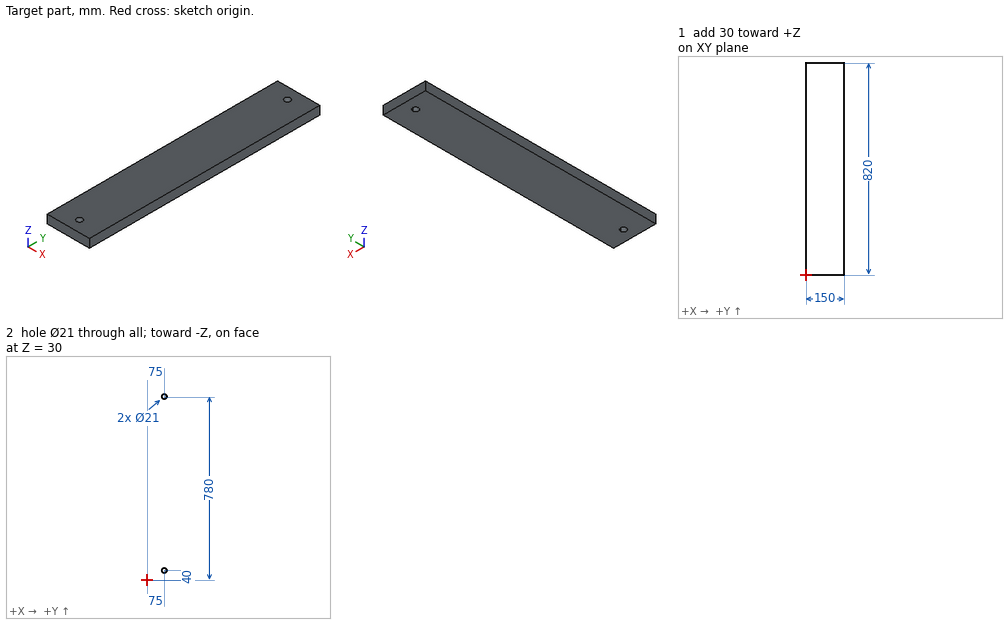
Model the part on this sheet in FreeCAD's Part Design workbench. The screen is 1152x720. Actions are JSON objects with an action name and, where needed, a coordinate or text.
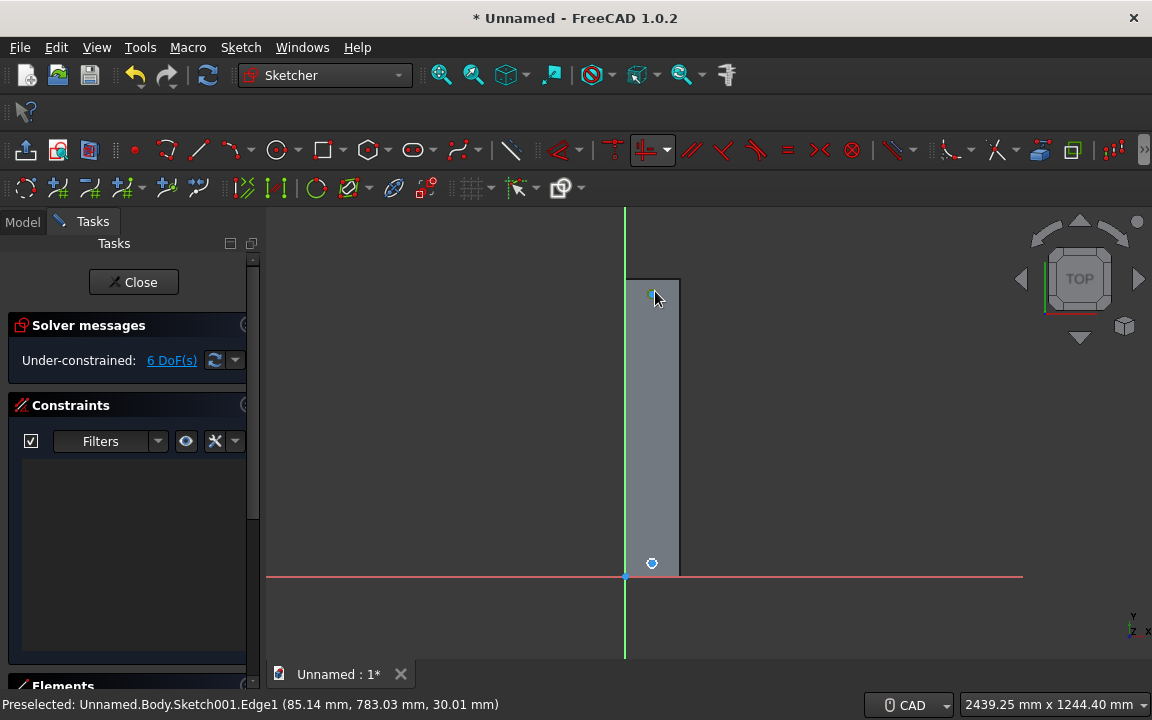
{"action": "scroll", "coordinate": [655, 560], "scroll_direction": "up", "scroll_amount": 6}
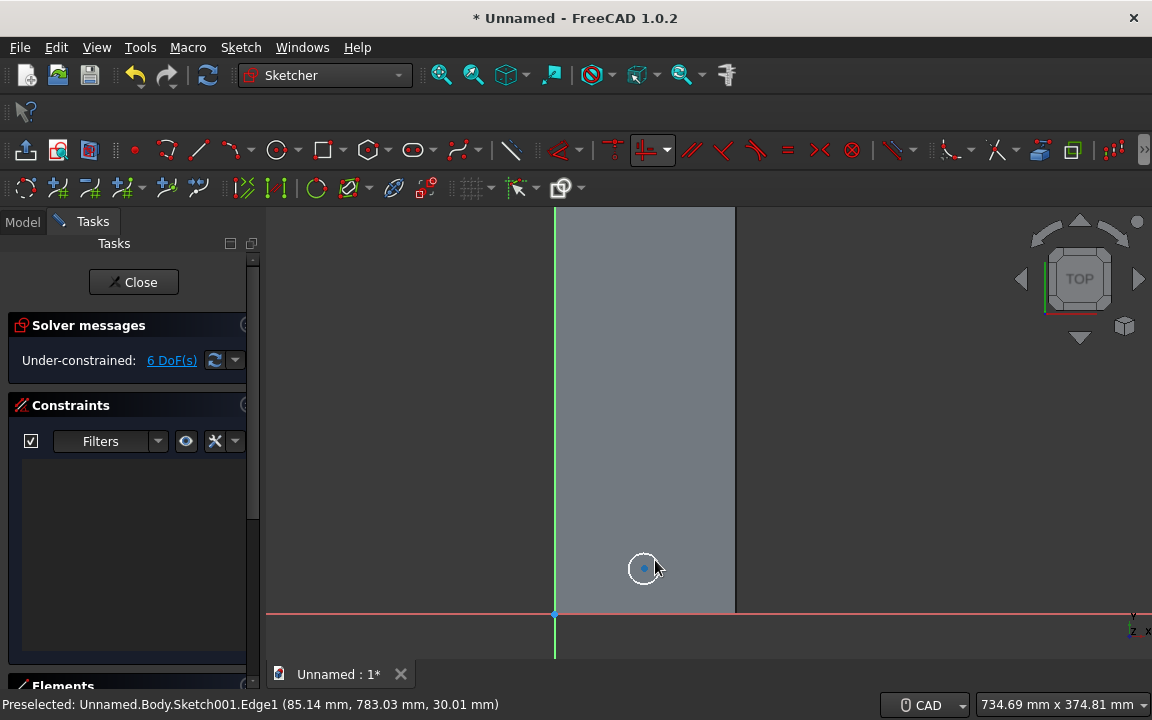
{"action": "left_click", "coordinate": [655, 558]}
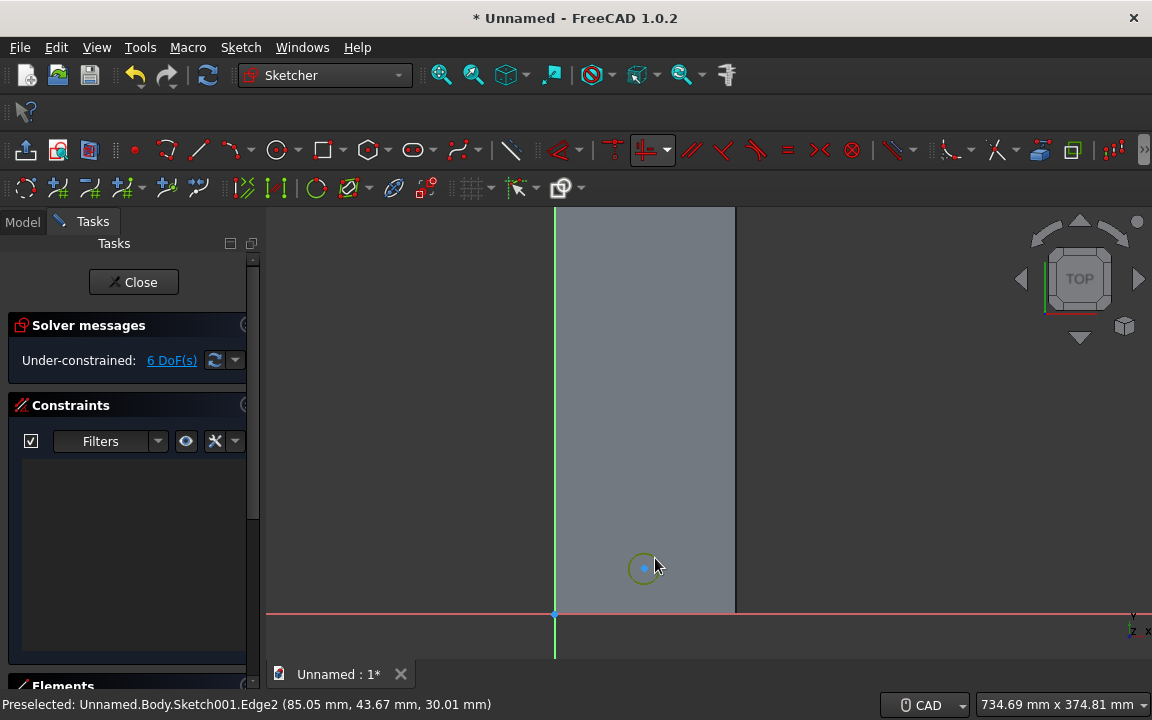
{"action": "left_click", "coordinate": [788, 150]}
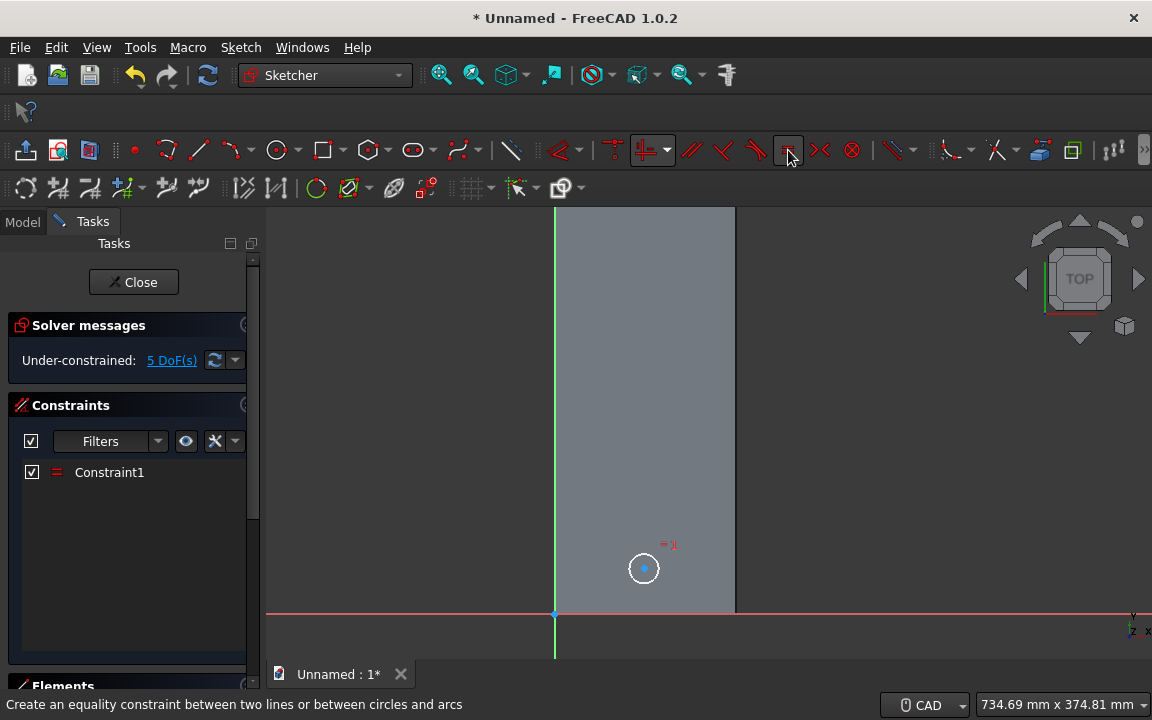
{"action": "left_click", "coordinate": [558, 150]}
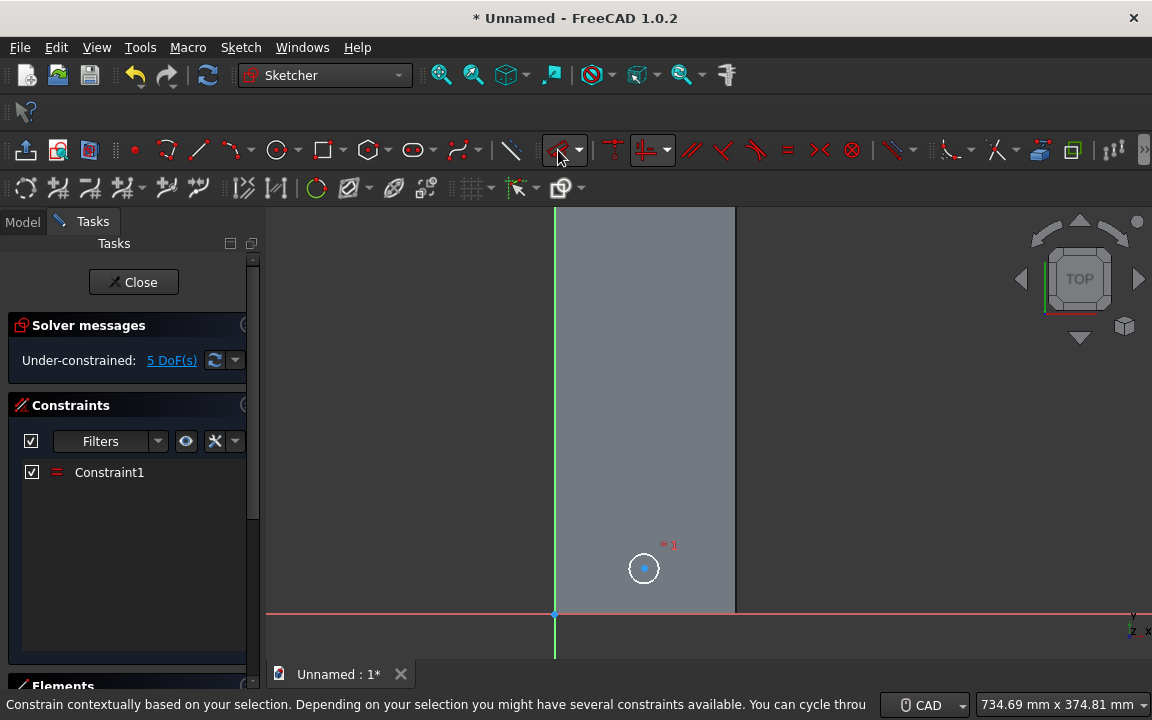
{"action": "scroll", "coordinate": [655, 560], "scroll_direction": "down", "scroll_amount": 6}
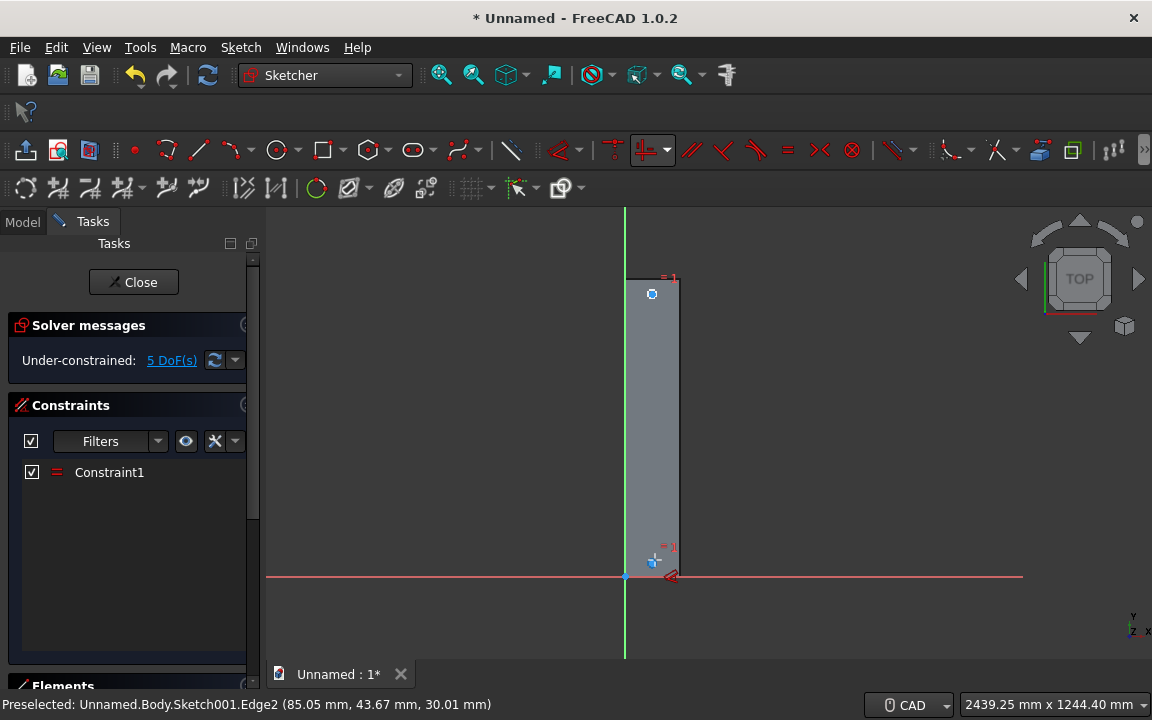
{"action": "scroll", "coordinate": [655, 291], "scroll_direction": "up", "scroll_amount": 9}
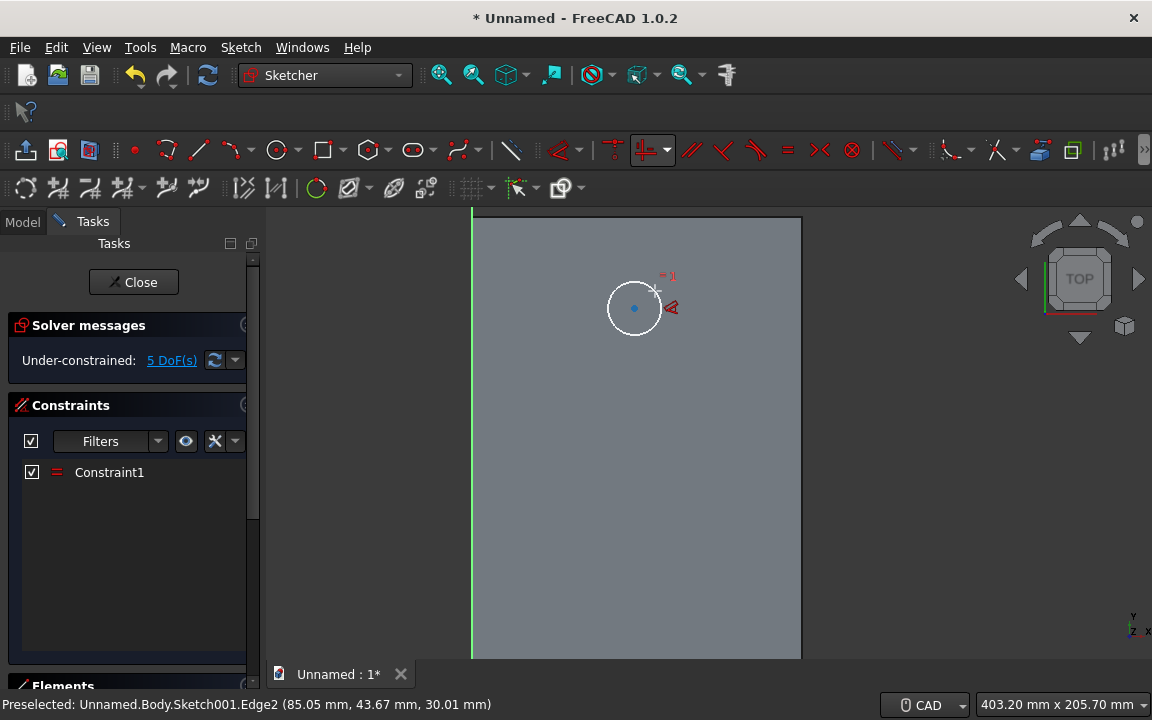
{"action": "left_click", "coordinate": [653, 290]}
{"action": "left_click", "coordinate": [676, 267]}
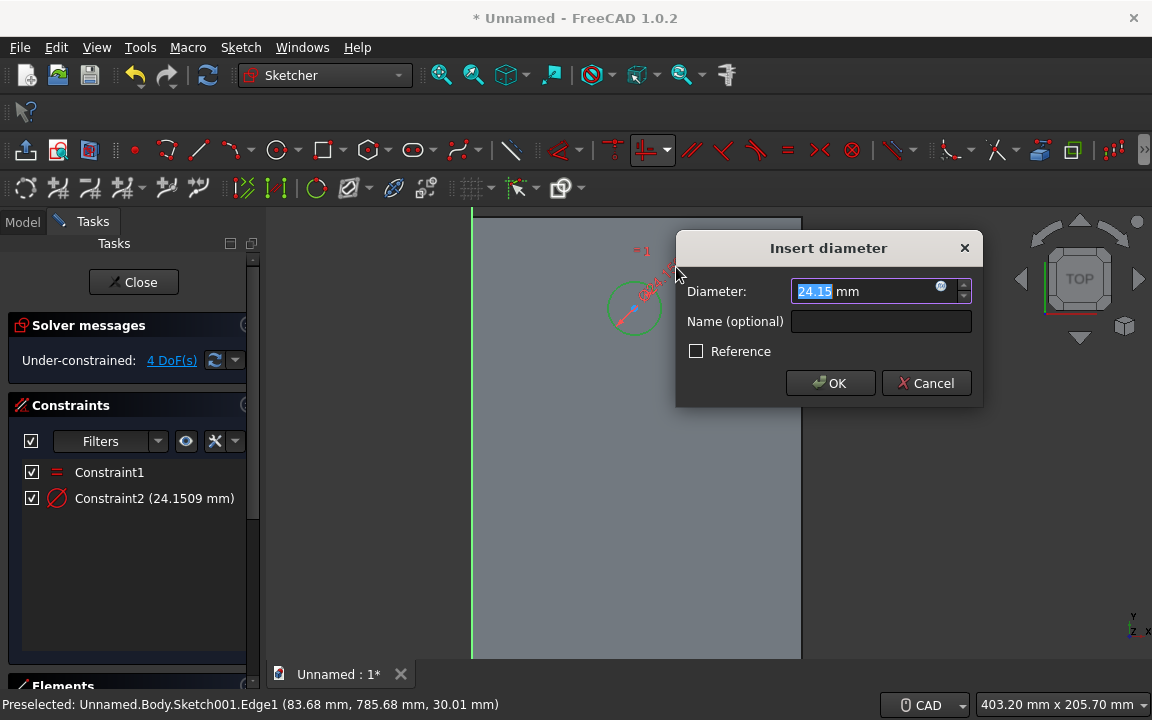
{"action": "type", "text": "21"}
{"action": "key", "text": "Return"}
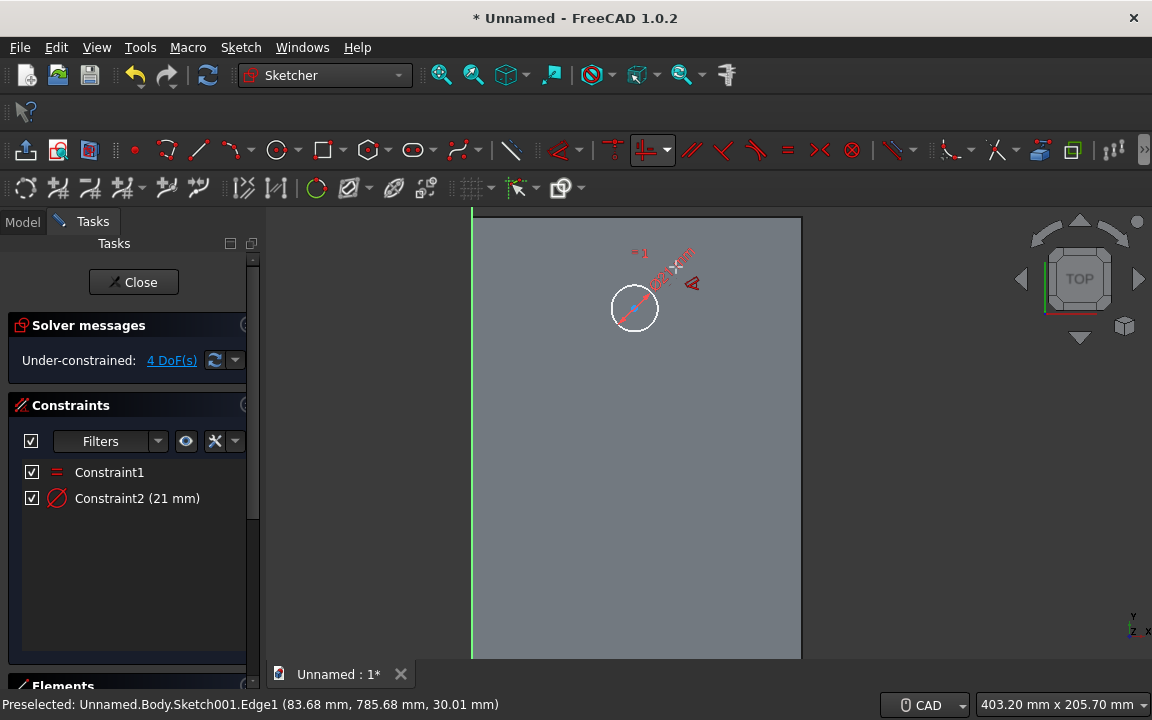
{"action": "scroll", "coordinate": [655, 291], "scroll_direction": "down", "scroll_amount": 9}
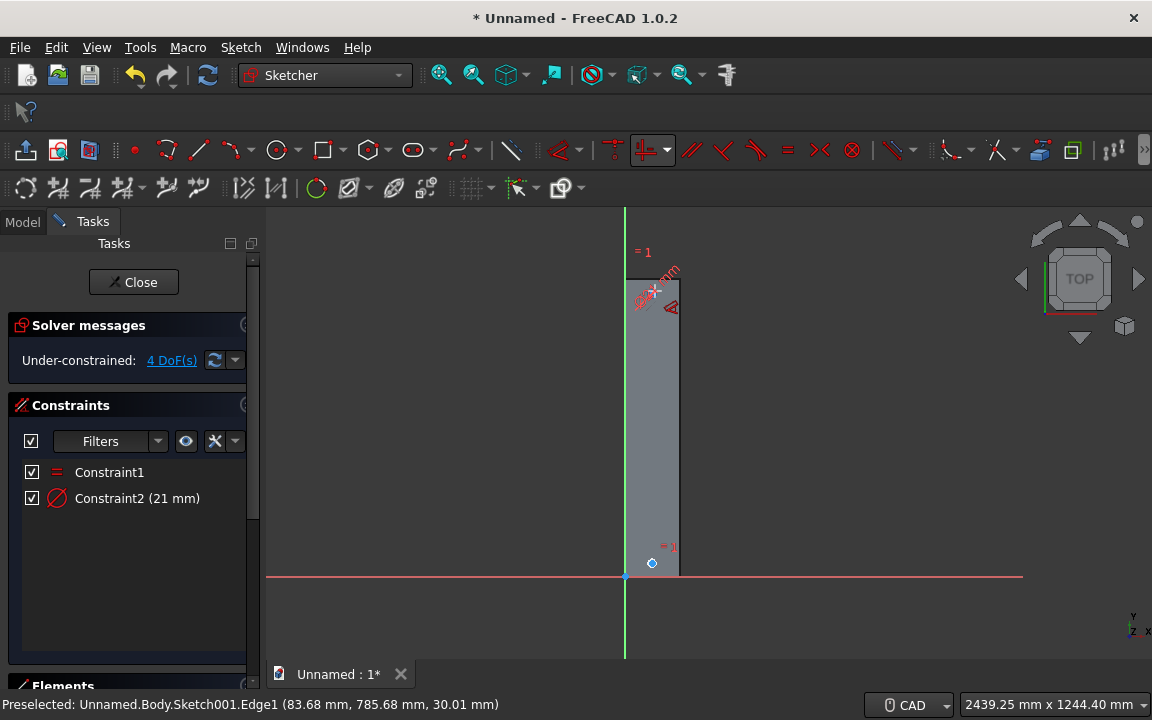
{"action": "scroll", "coordinate": [652, 294], "scroll_direction": "up", "scroll_amount": 2}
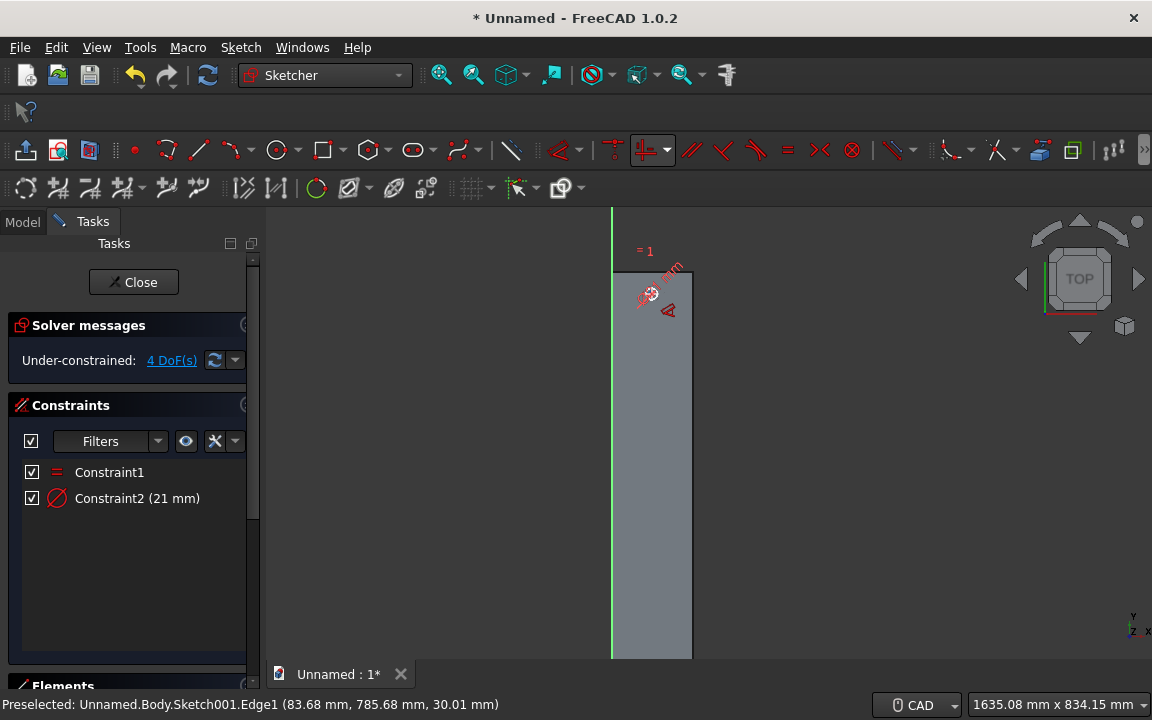
{"action": "left_click", "coordinate": [652, 294]}
{"action": "left_click", "coordinate": [632, 260]}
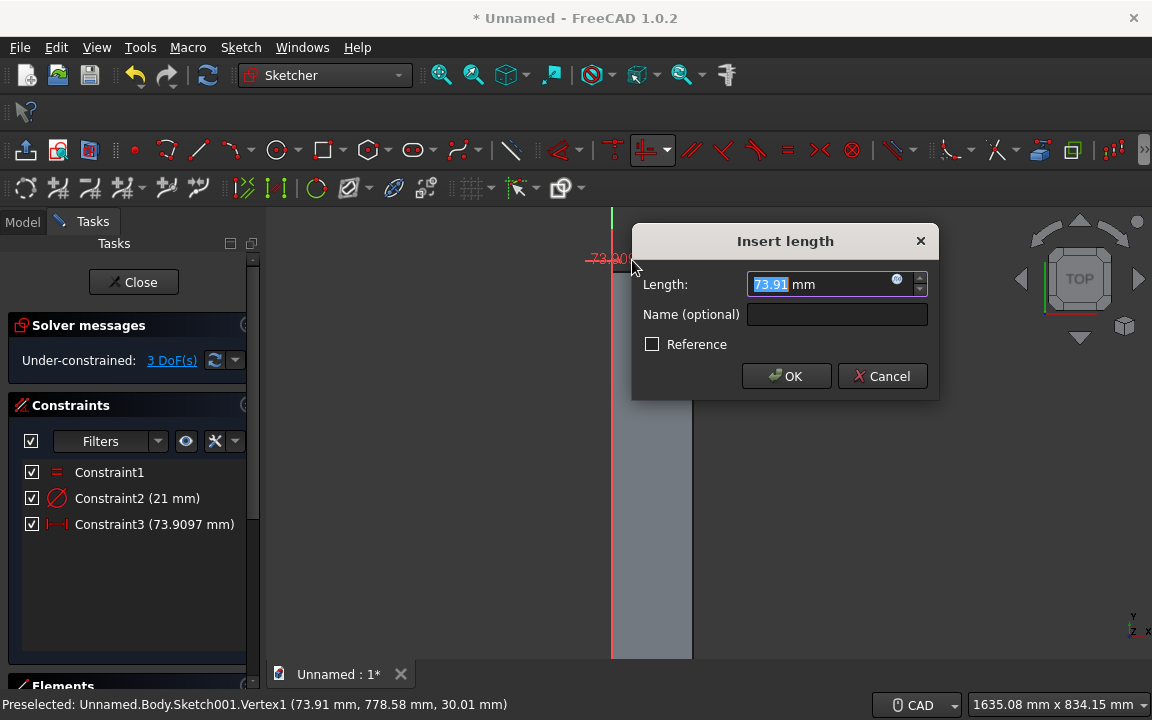
{"action": "type", "text": "75"}
{"action": "key", "text": "Return"}